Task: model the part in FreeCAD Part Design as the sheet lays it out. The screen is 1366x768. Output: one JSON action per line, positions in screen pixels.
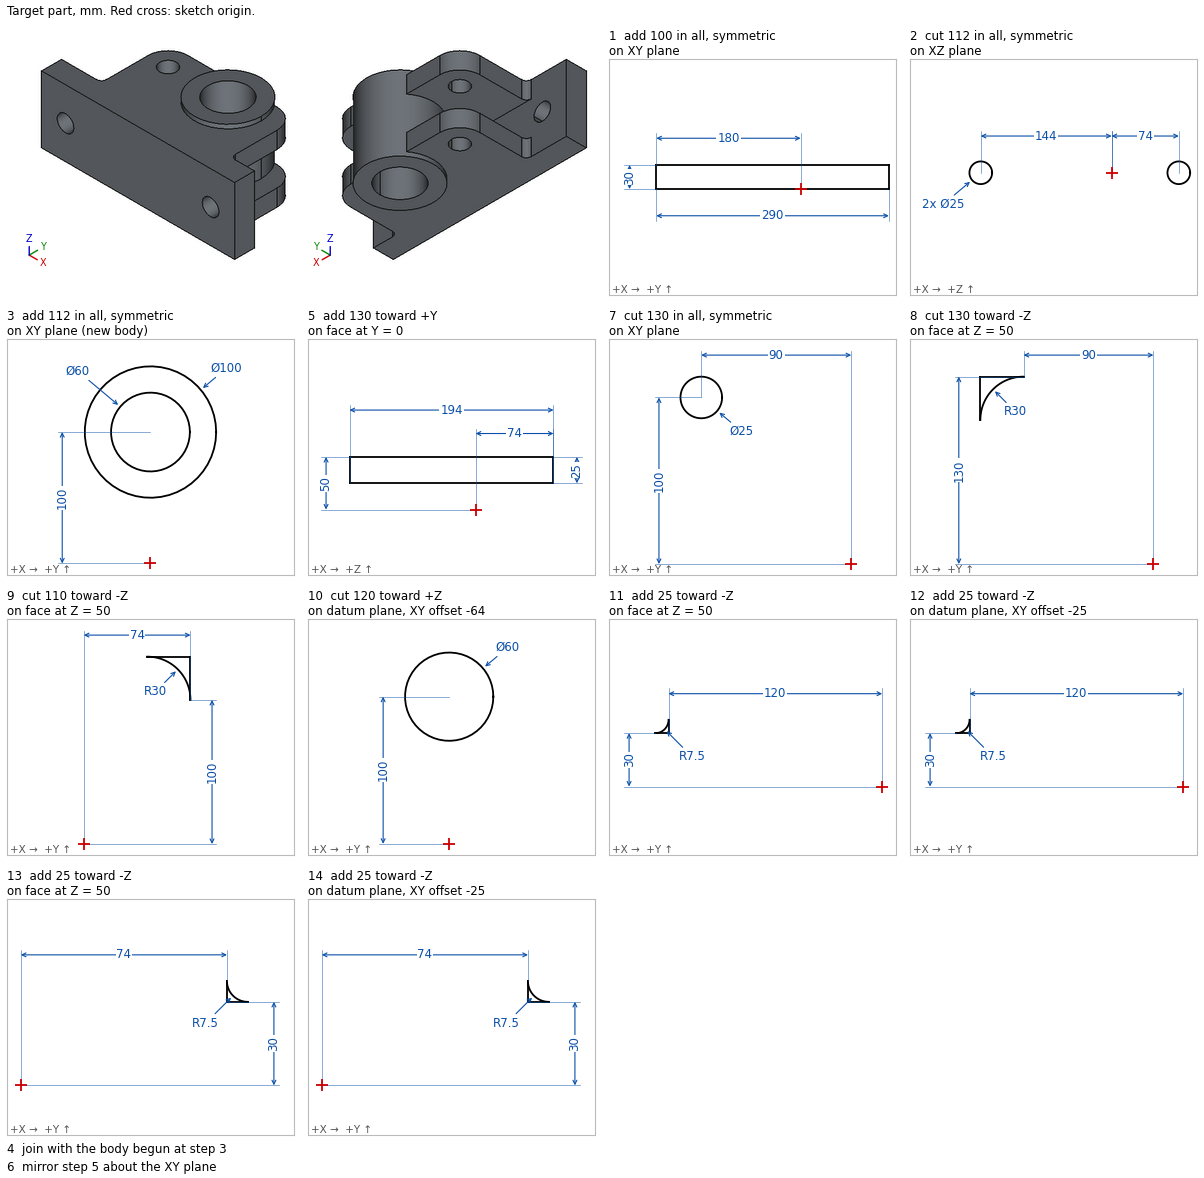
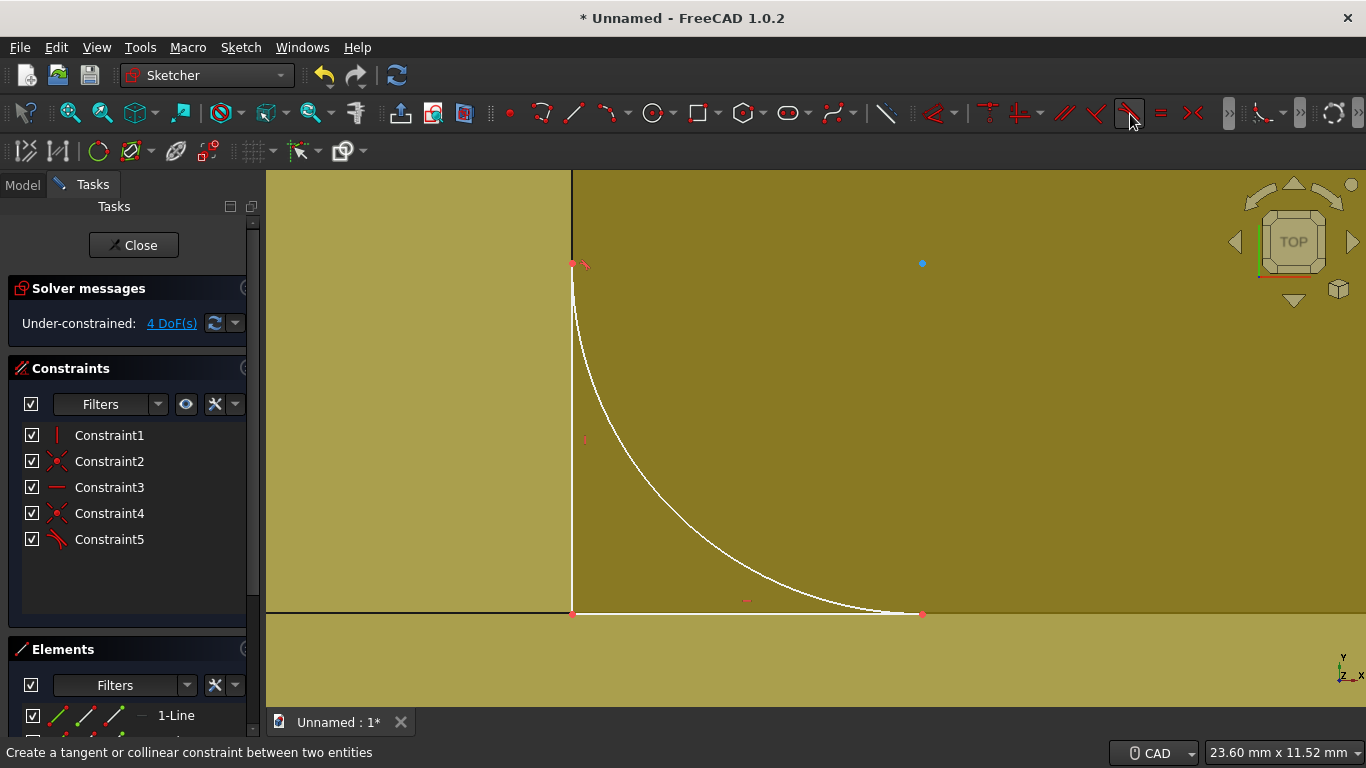
{"action": "left_click", "coordinate": [677, 614]}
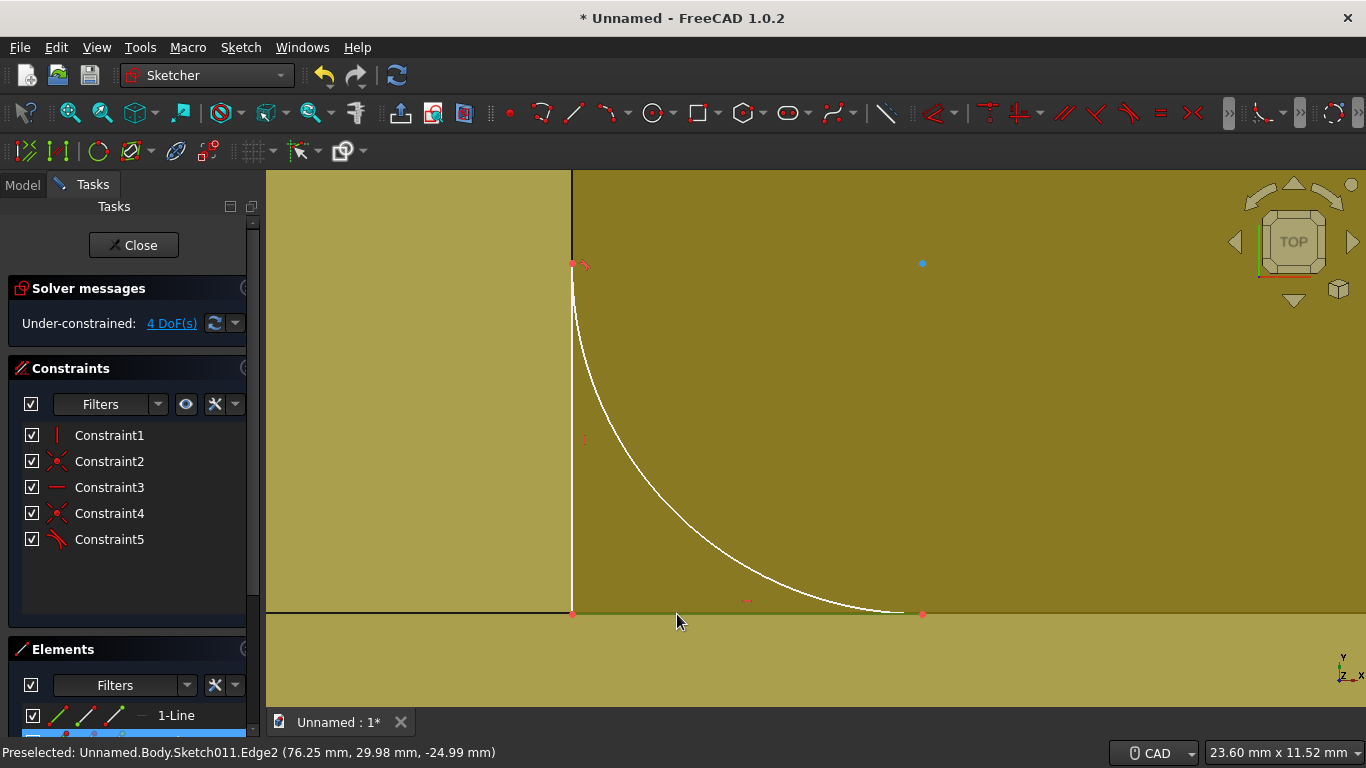
{"action": "left_click", "coordinate": [610, 423]}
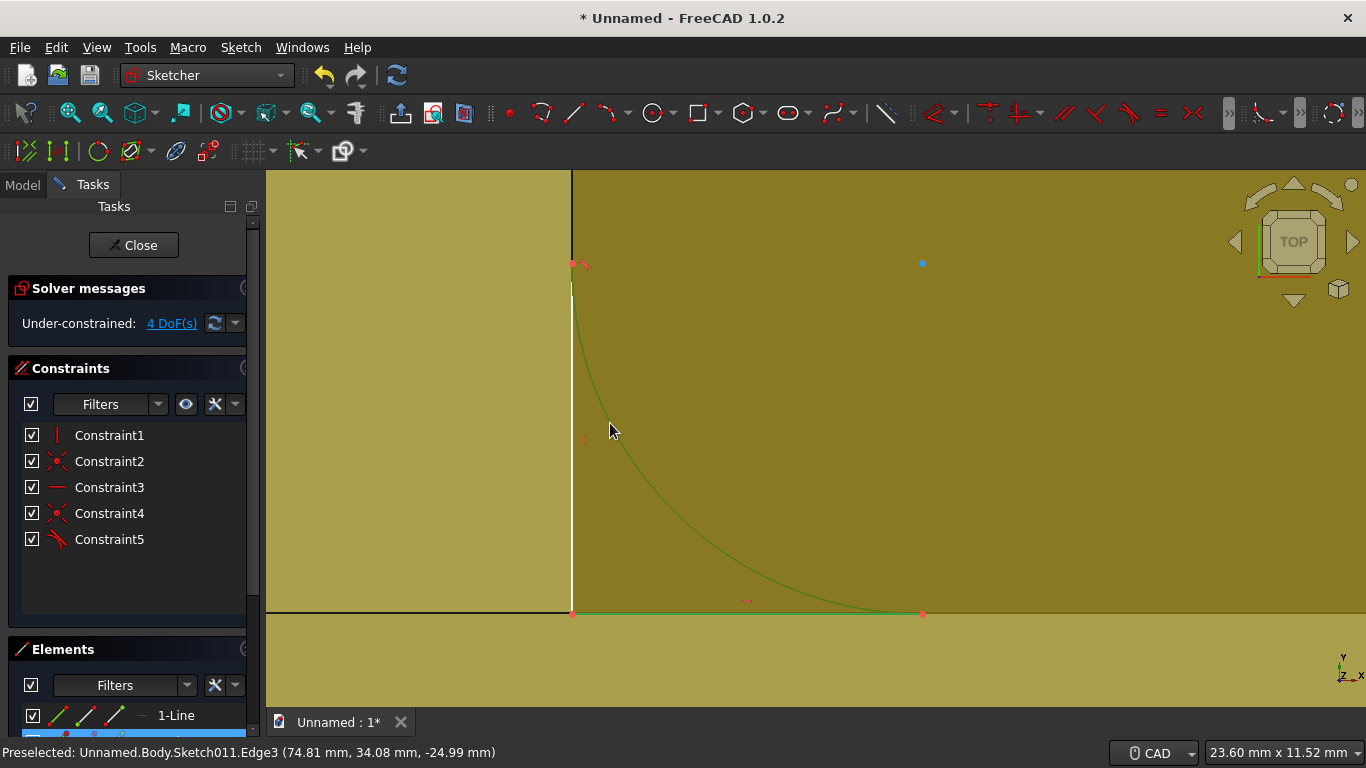
{"action": "left_click", "coordinate": [1130, 114]}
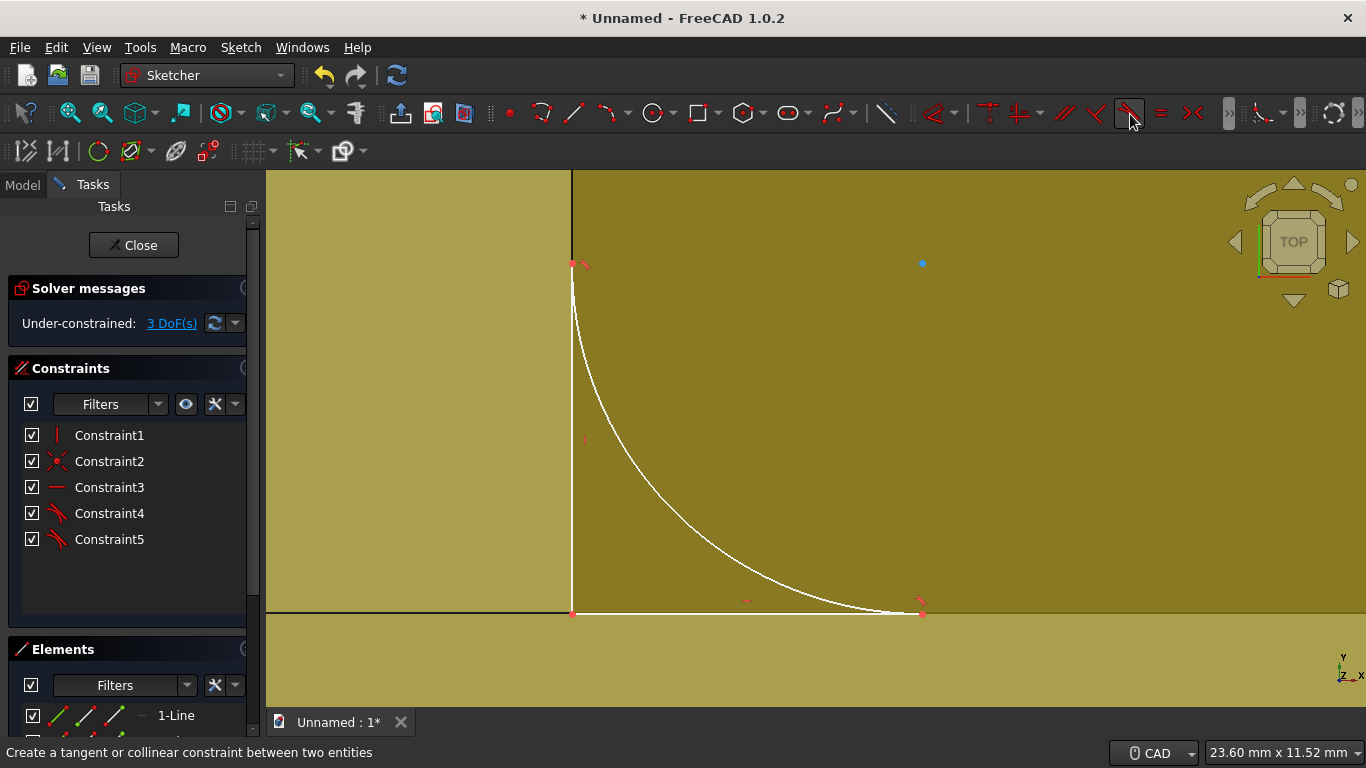
{"action": "left_click", "coordinate": [934, 114]}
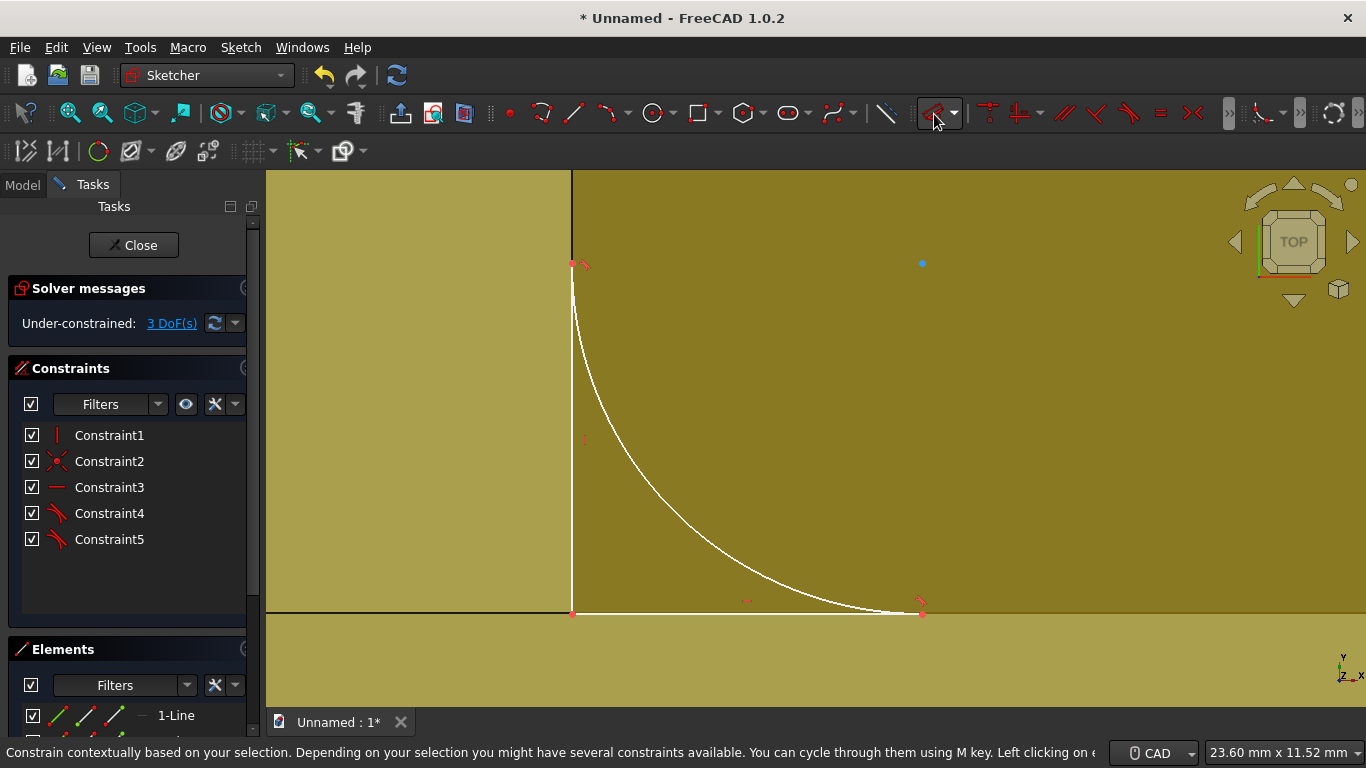
{"action": "left_click", "coordinate": [610, 423]}
{"action": "left_click", "coordinate": [540, 253]}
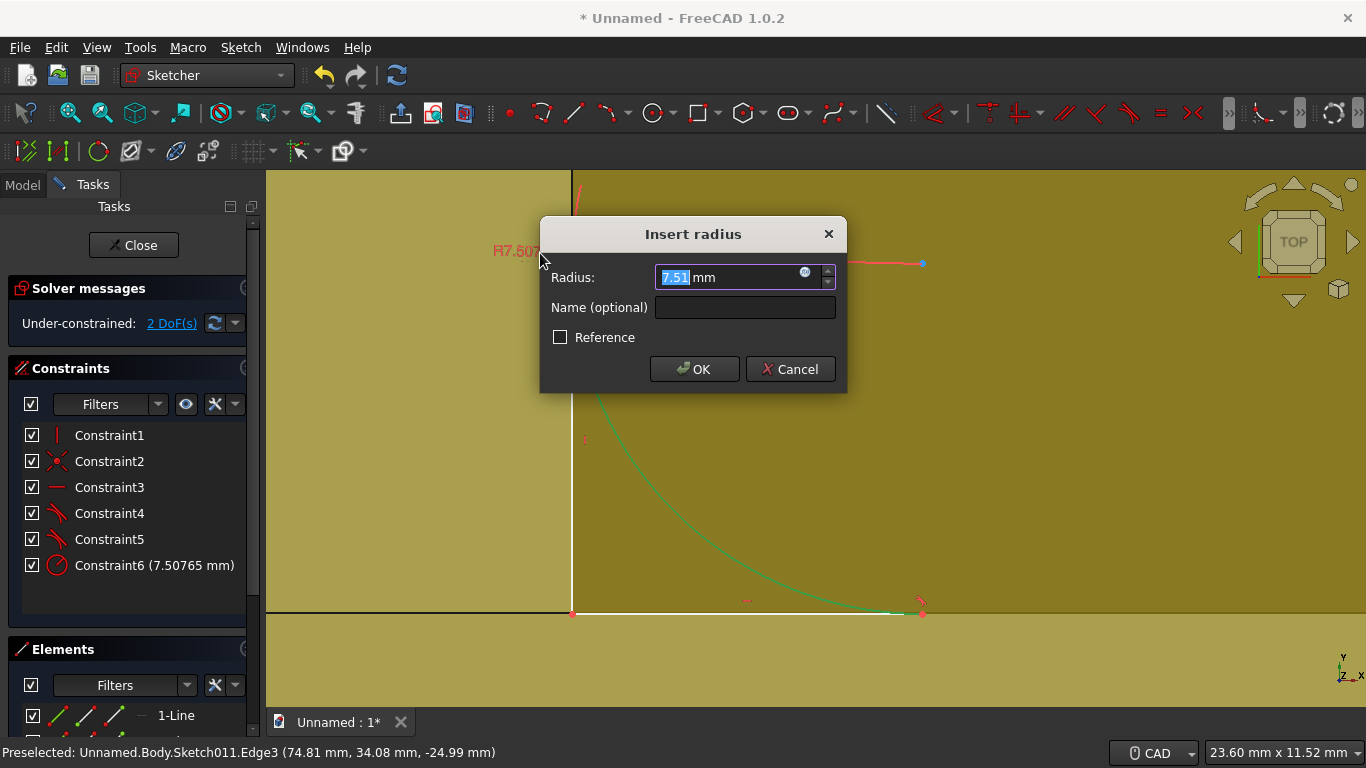
{"action": "type", "text": "7.5"}
{"action": "key", "text": "Return"}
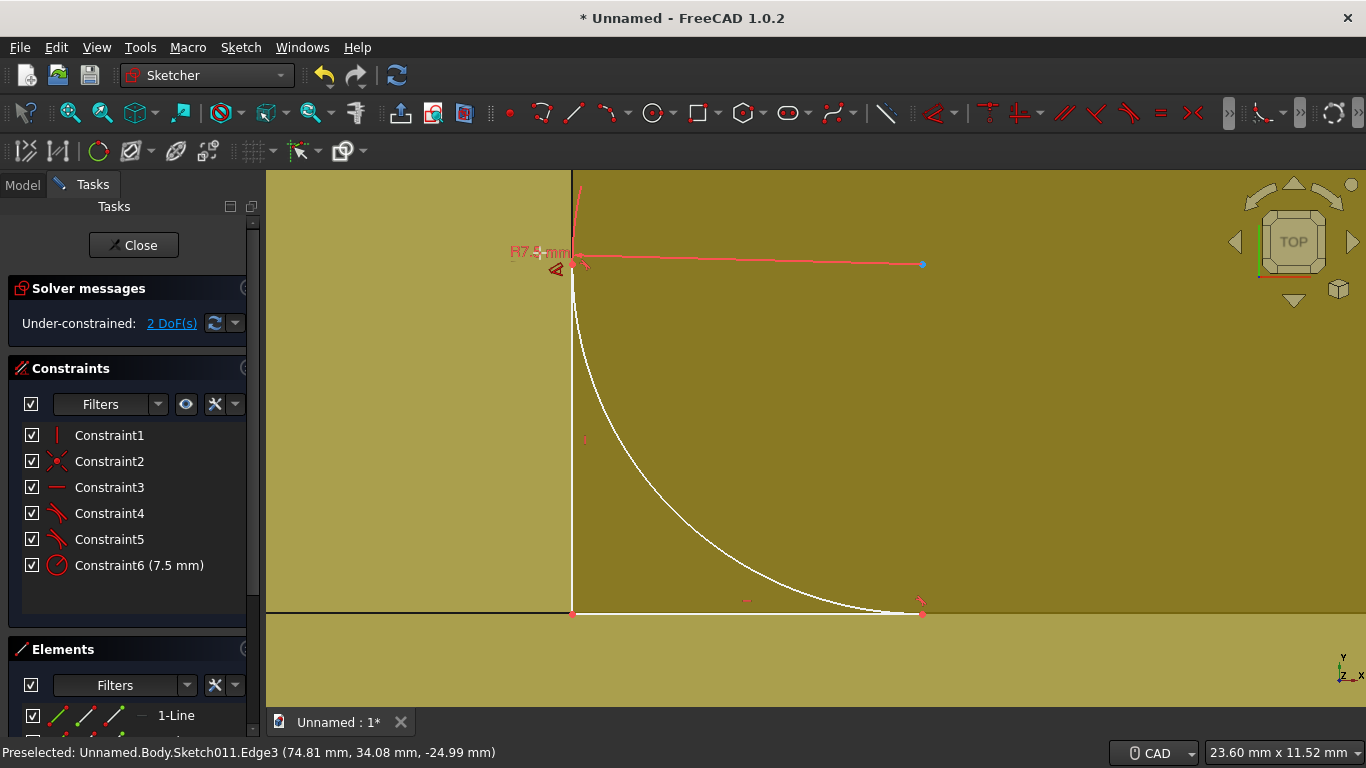
{"action": "left_click", "coordinate": [572, 264]}
{"action": "left_click", "coordinate": [433, 230]}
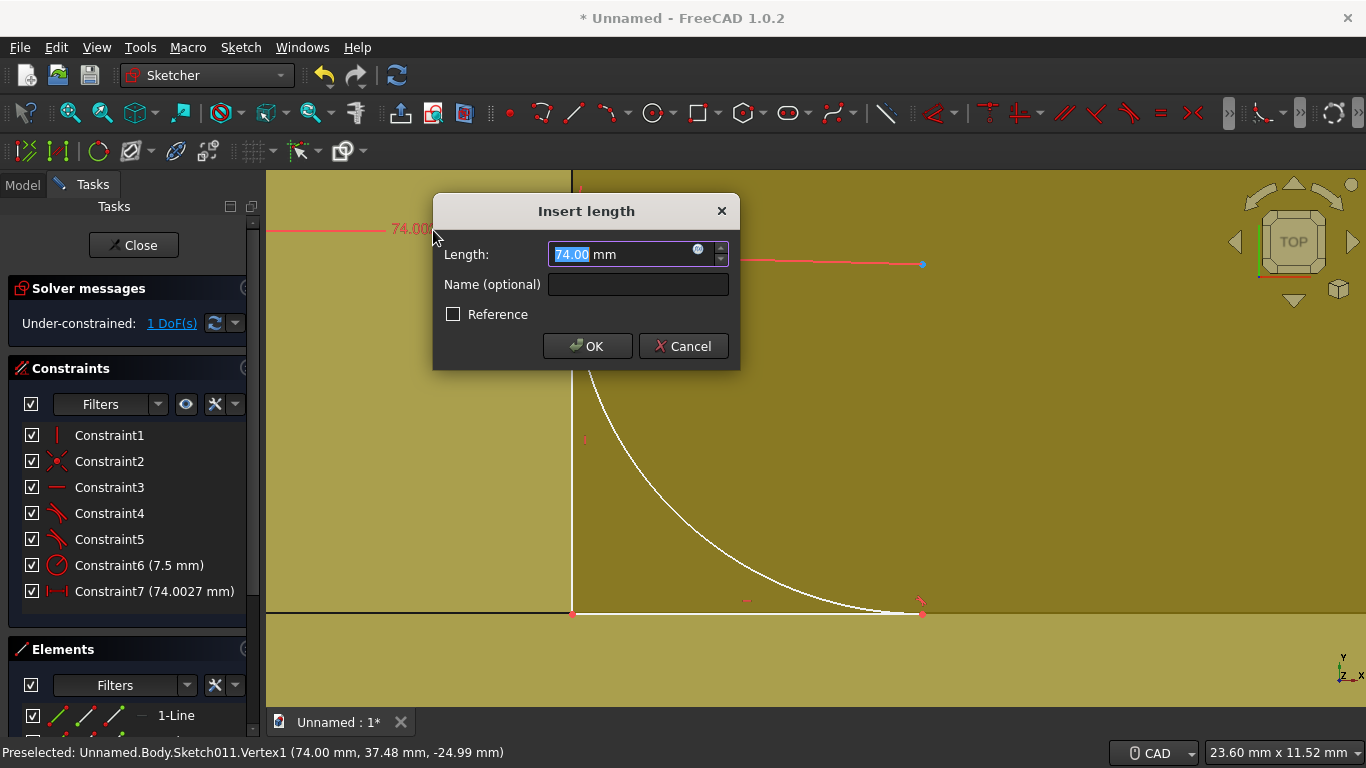
{"action": "type", "text": "74"}
{"action": "key", "text": "Return"}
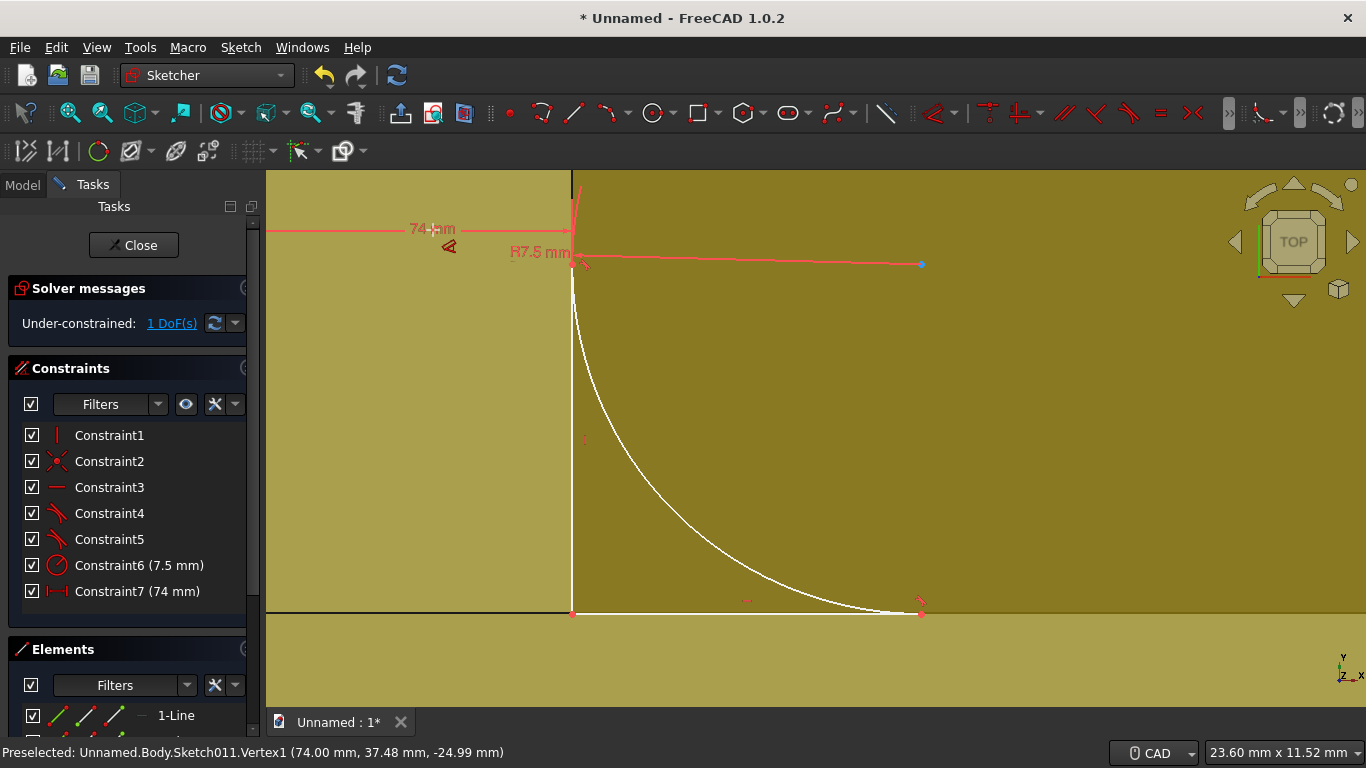
{"action": "left_click", "coordinate": [572, 614]}
{"action": "left_click", "coordinate": [606, 647]}